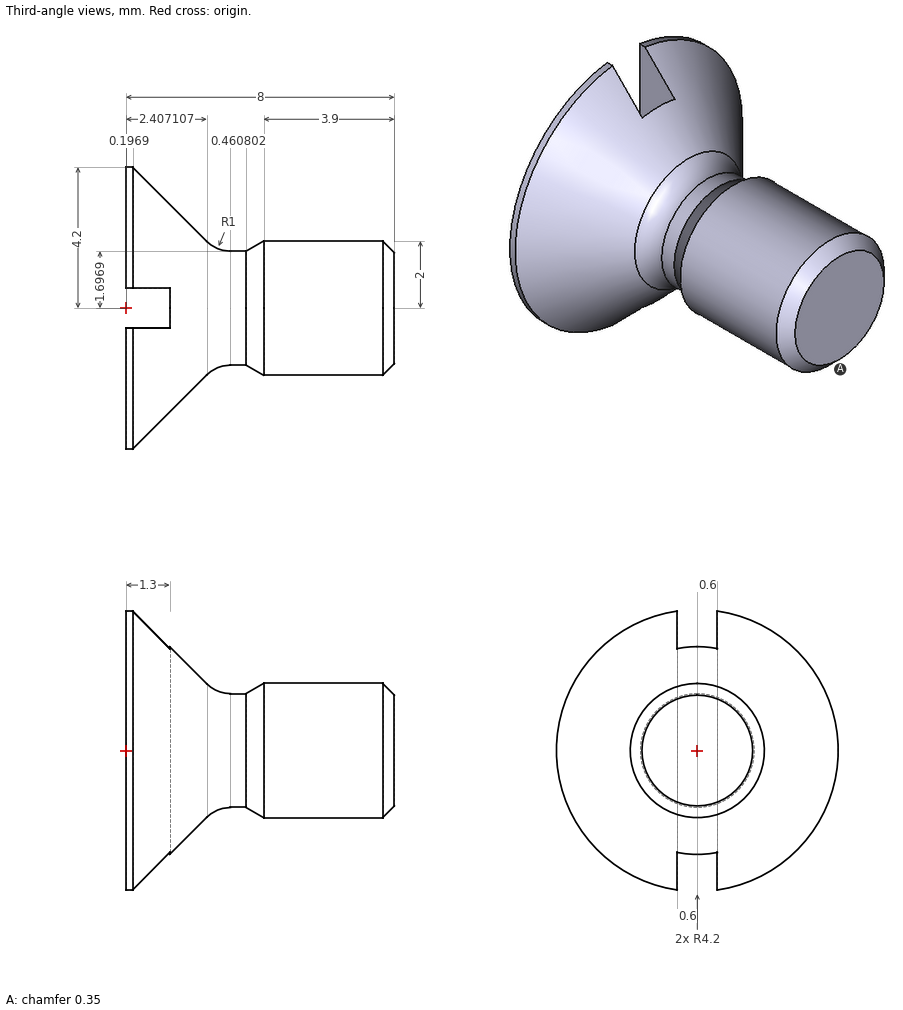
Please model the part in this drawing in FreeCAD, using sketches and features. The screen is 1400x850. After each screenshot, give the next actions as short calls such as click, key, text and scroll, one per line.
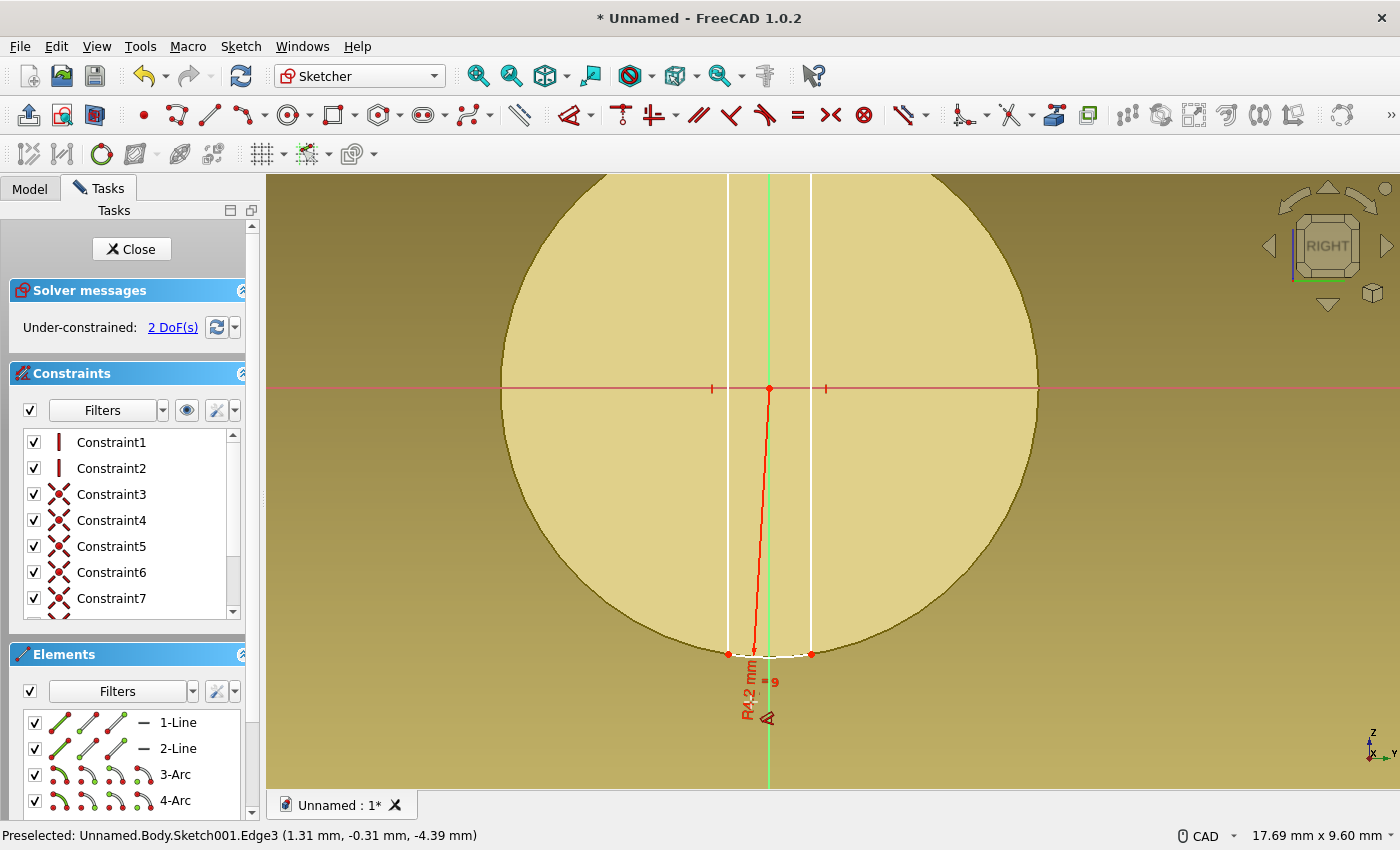
scroll(754, 671, down, 2)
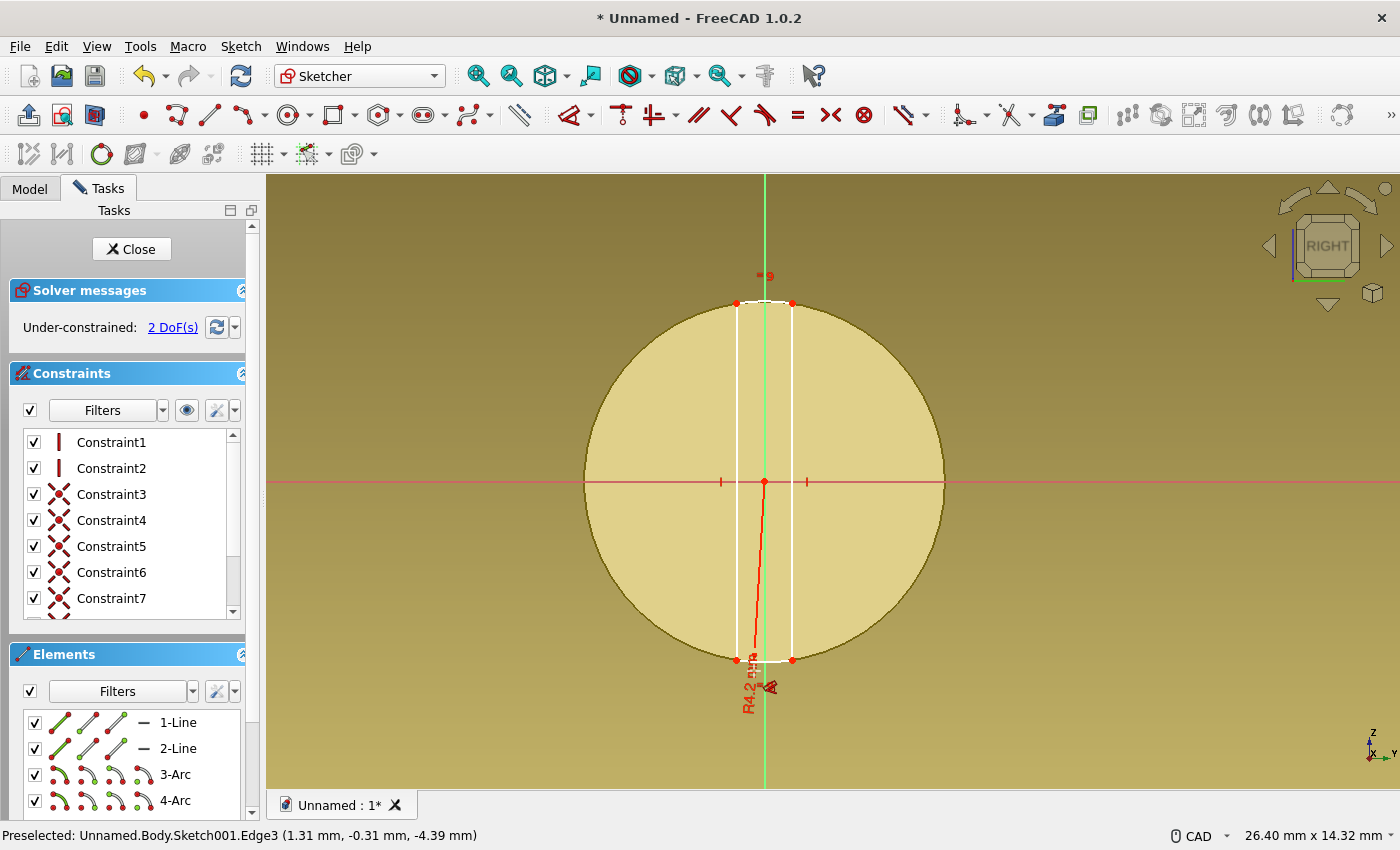
scroll(792, 304, up, 3)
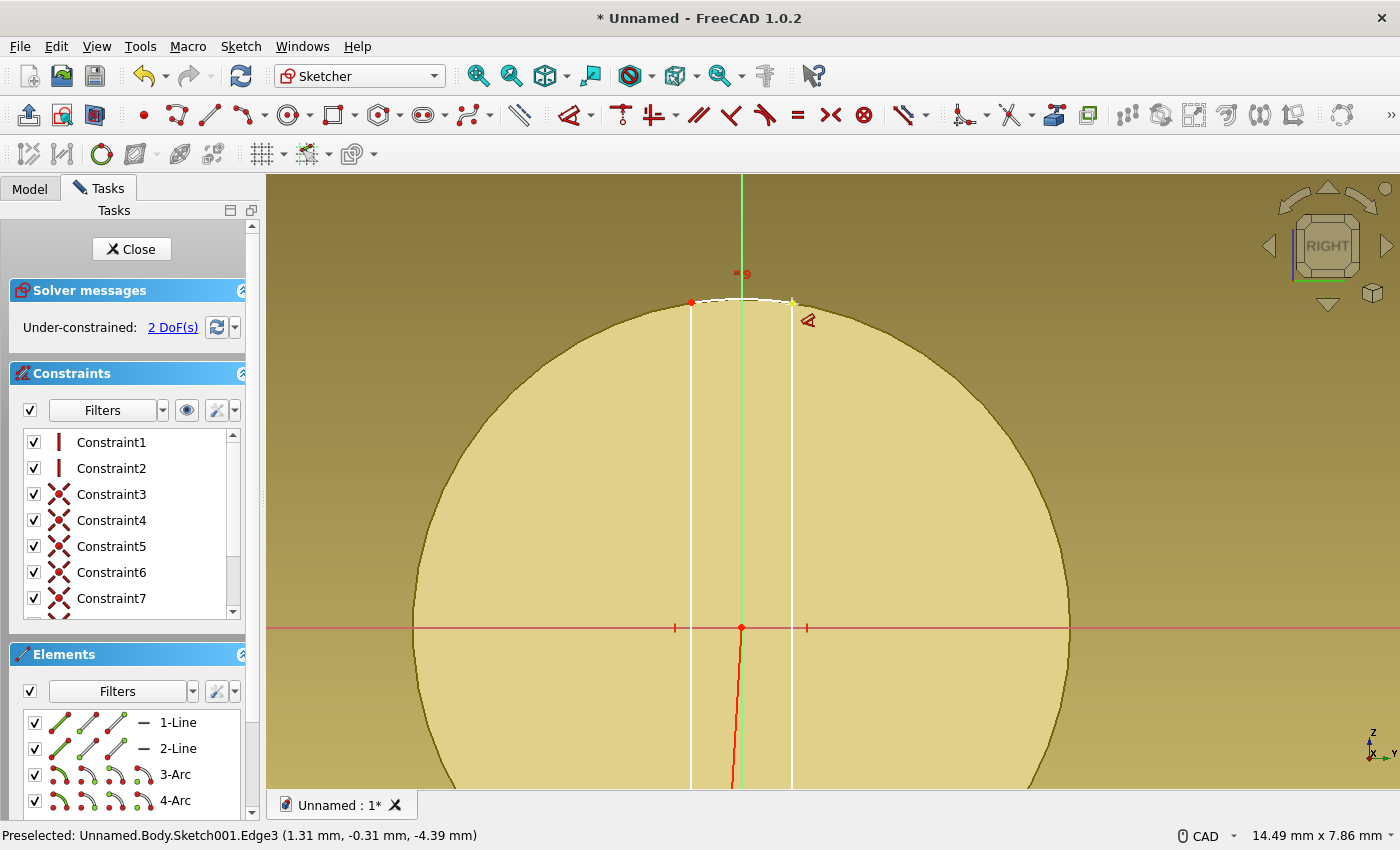
click(792, 303)
click(767, 269)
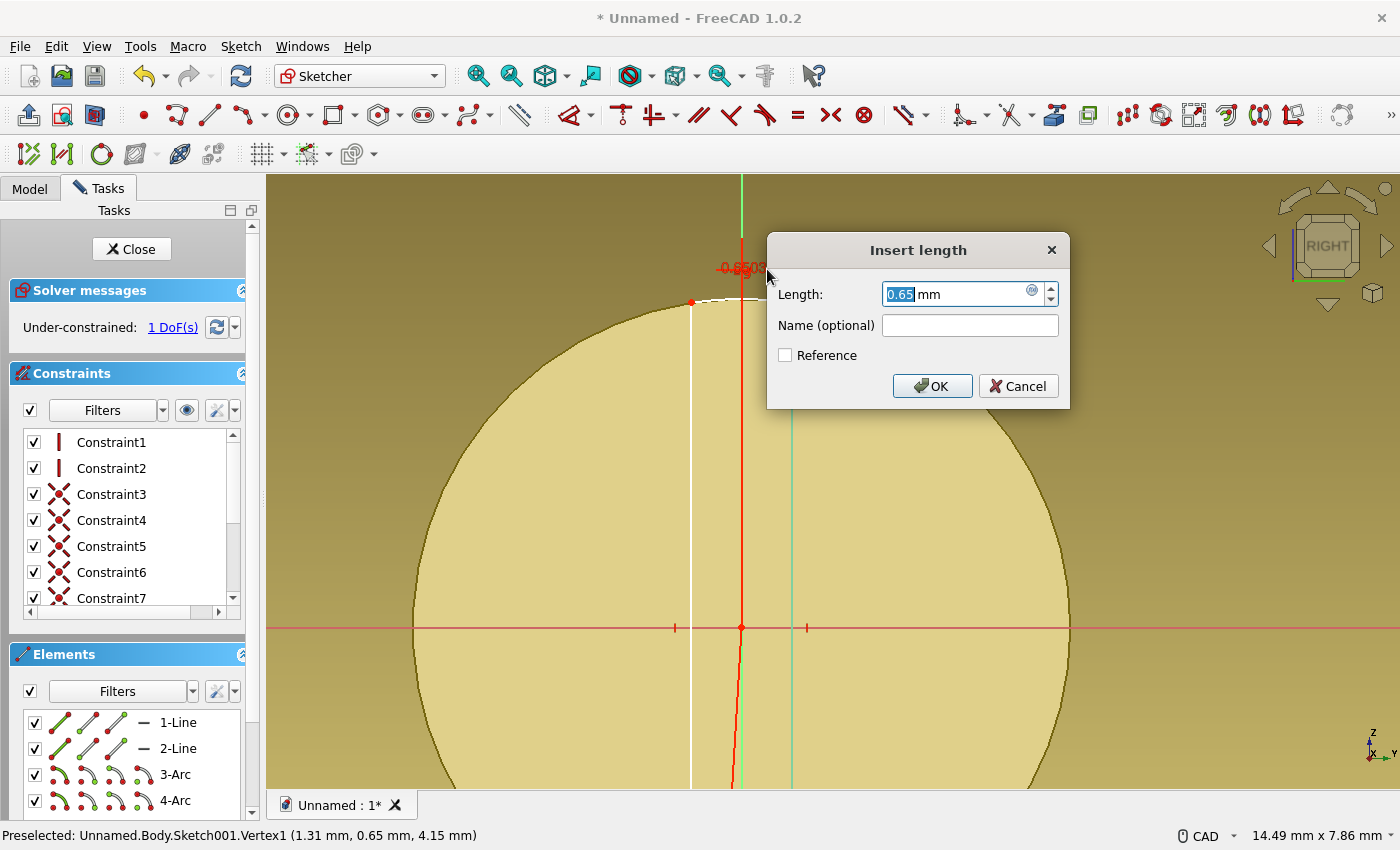
text(0.6)
key(Return)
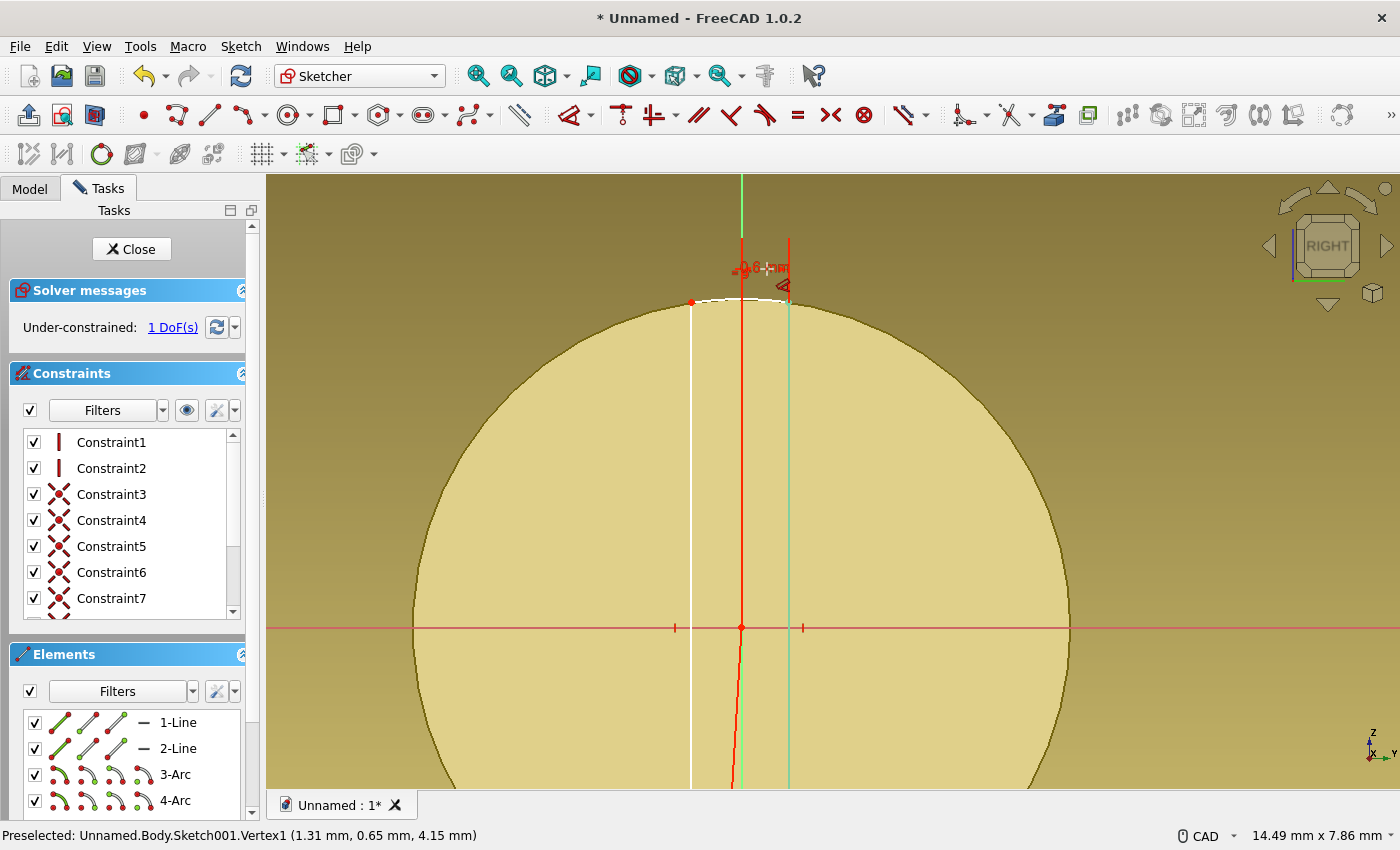
scroll(792, 303, down, 3)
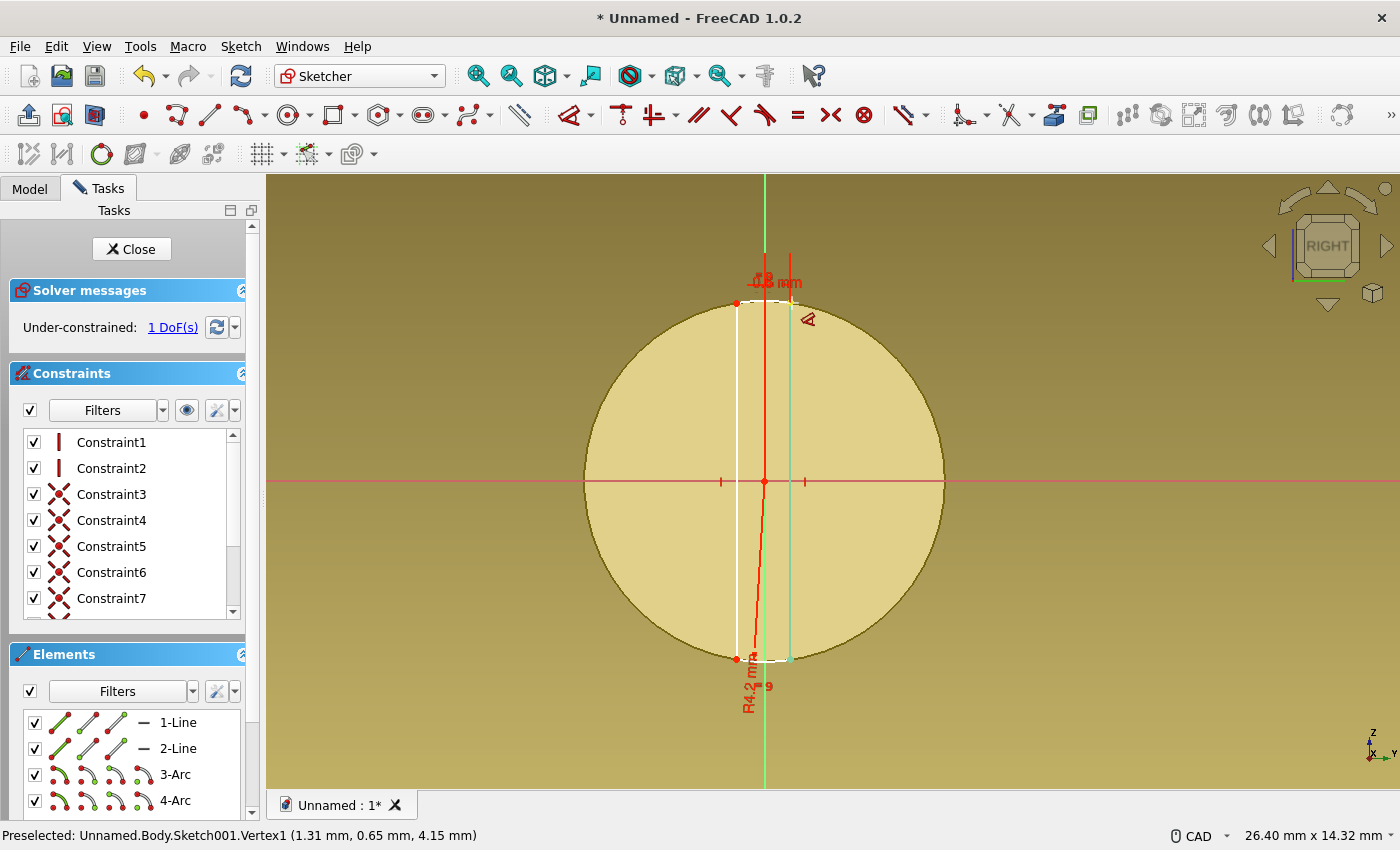
scroll(737, 660, up, 3)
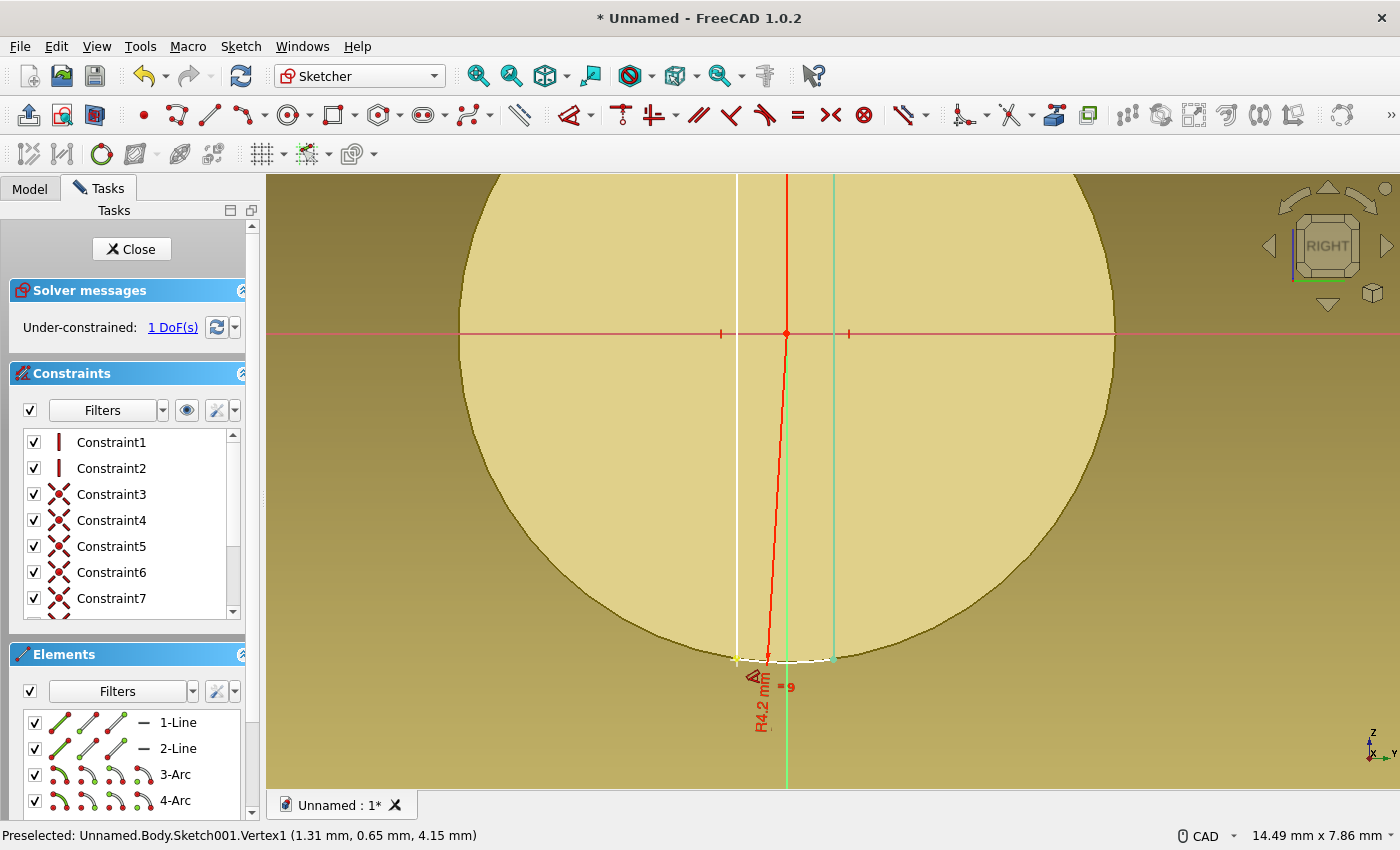
click(737, 659)
click(762, 693)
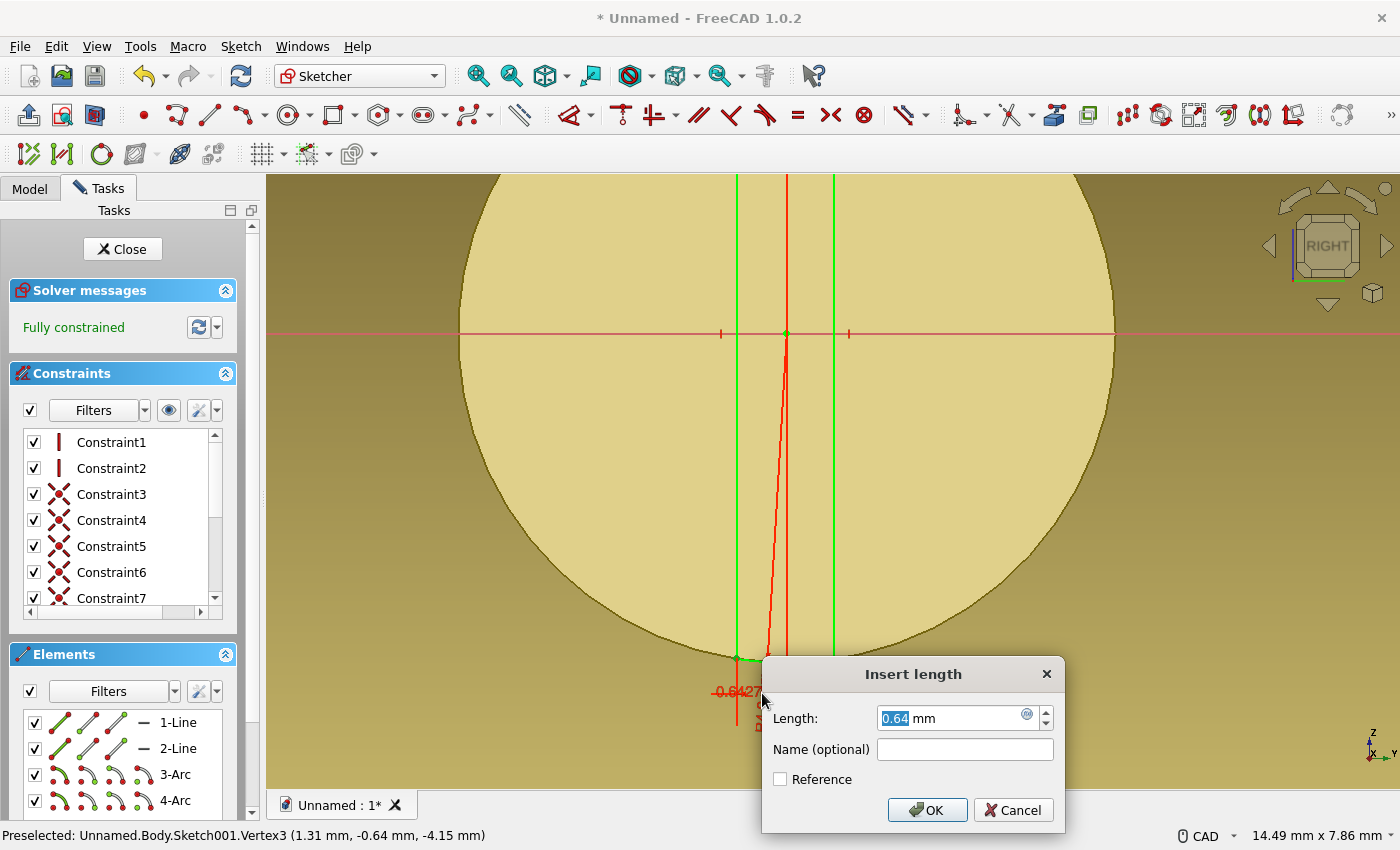
text(0.6)
key(Return)
key(Escape)